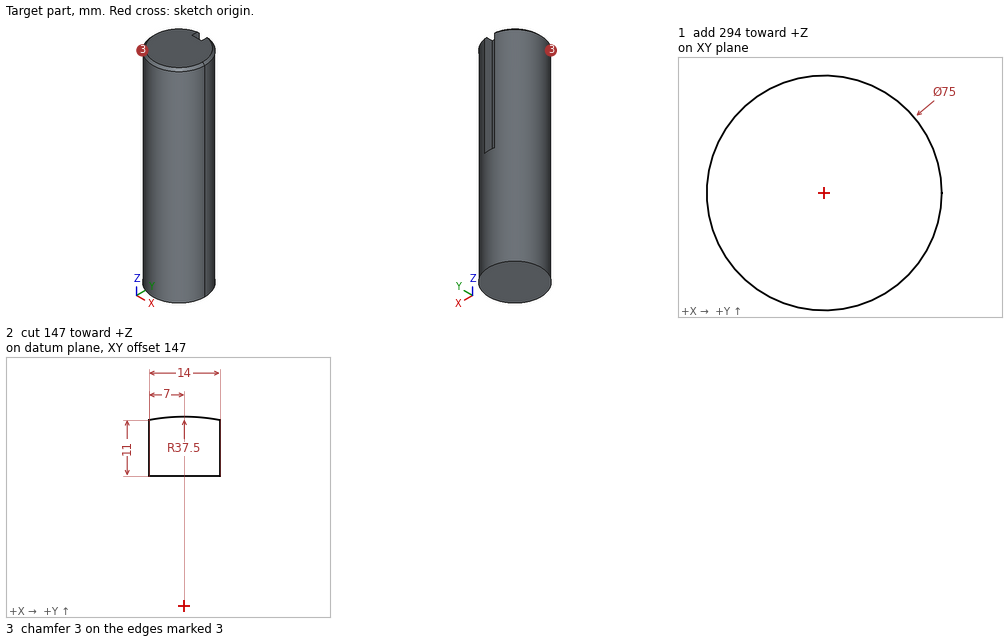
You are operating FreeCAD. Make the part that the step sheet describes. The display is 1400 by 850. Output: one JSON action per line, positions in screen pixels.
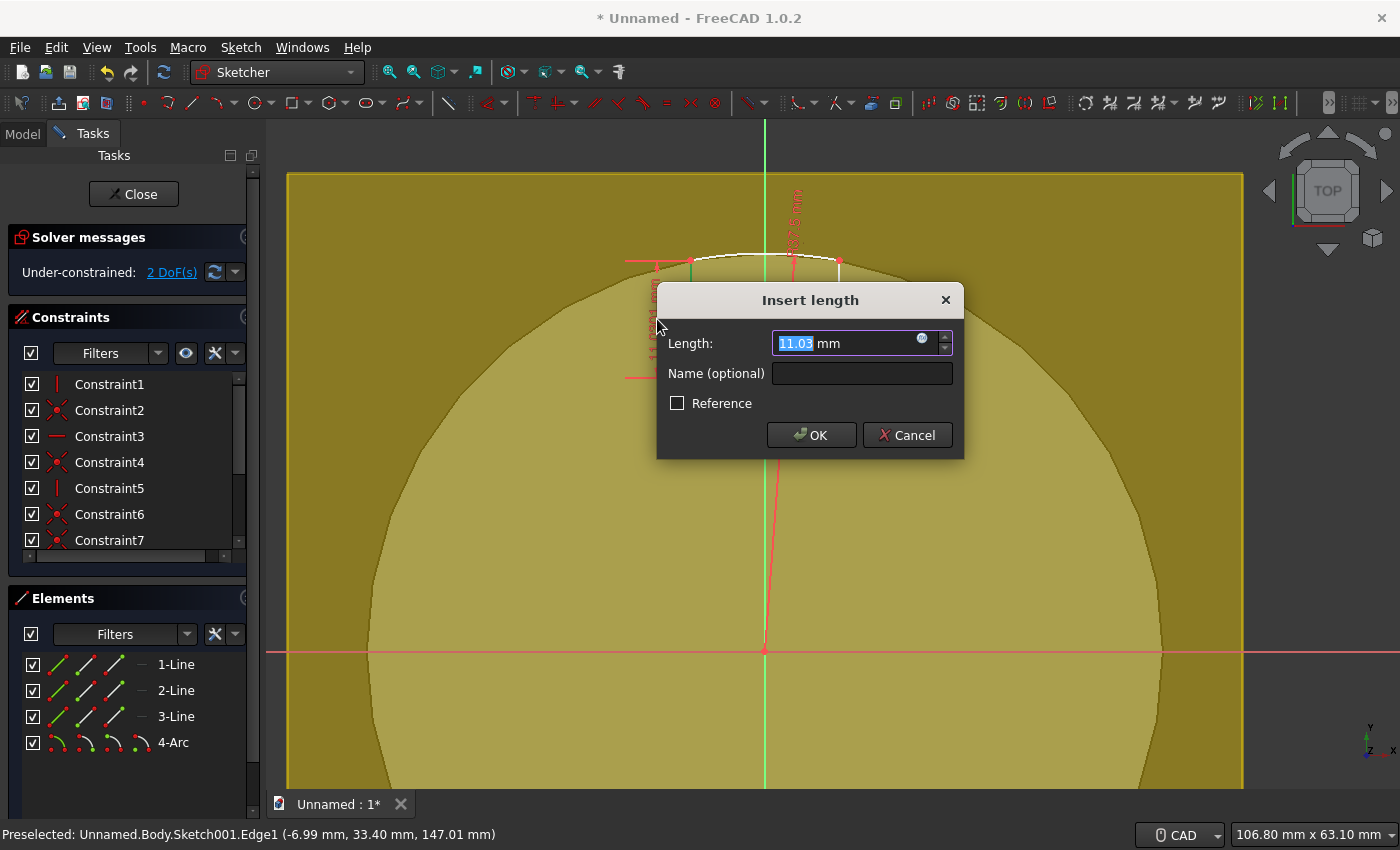
{"action": "type", "text": "11"}
{"action": "key", "text": "Return"}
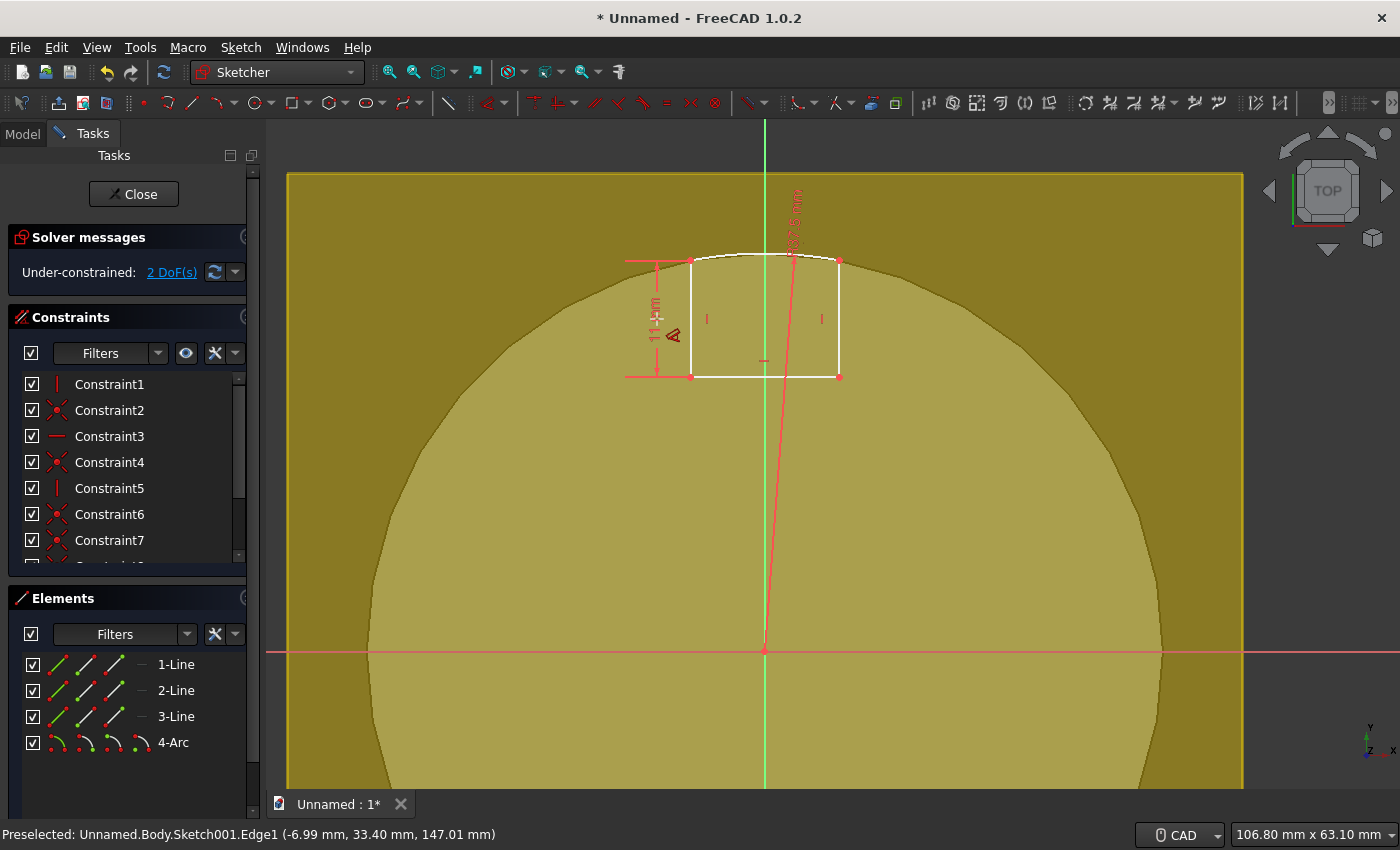
{"action": "left_click", "coordinate": [735, 377]}
{"action": "left_click", "coordinate": [731, 411]}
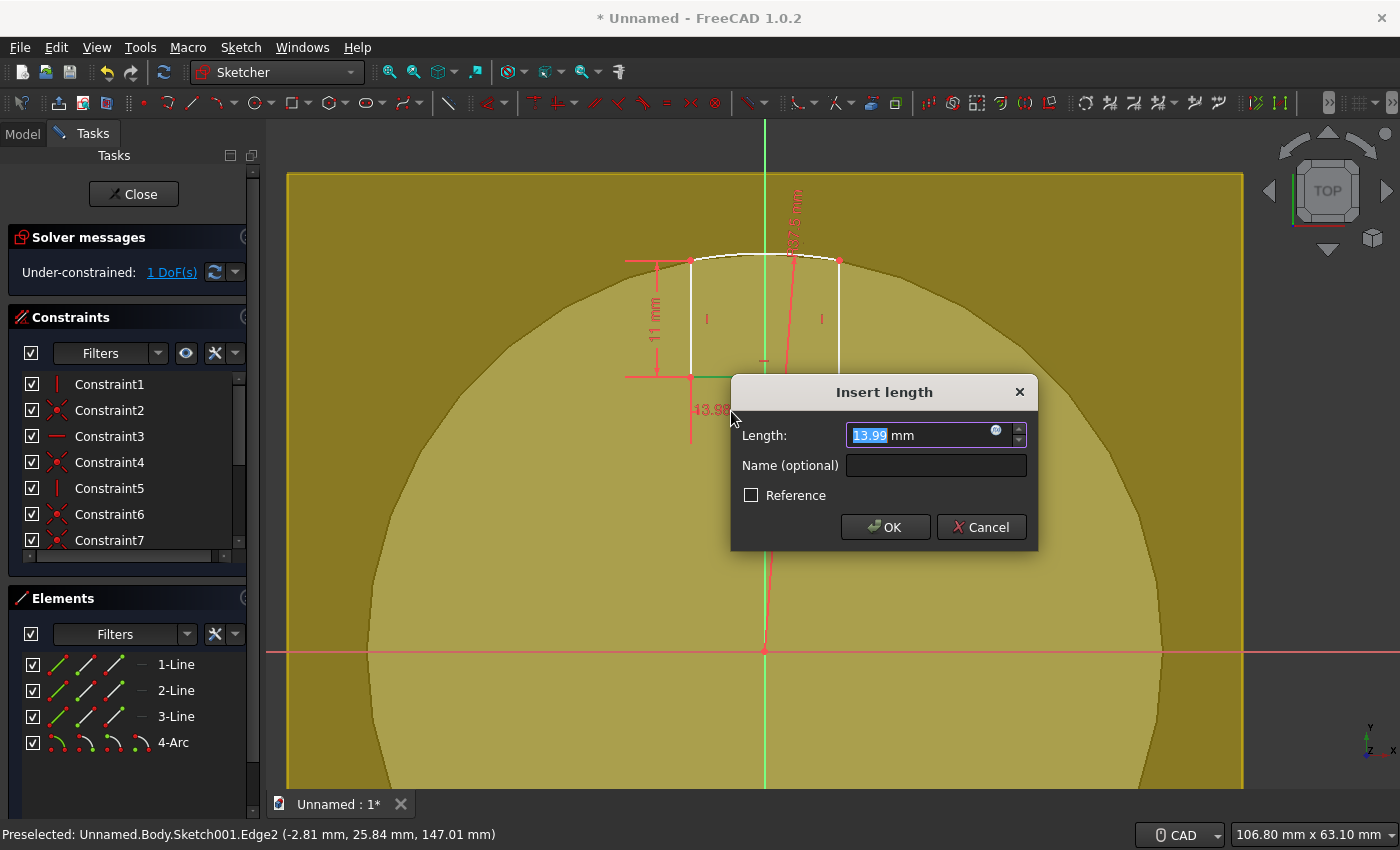
{"action": "type", "text": "14"}
{"action": "key", "text": "Return"}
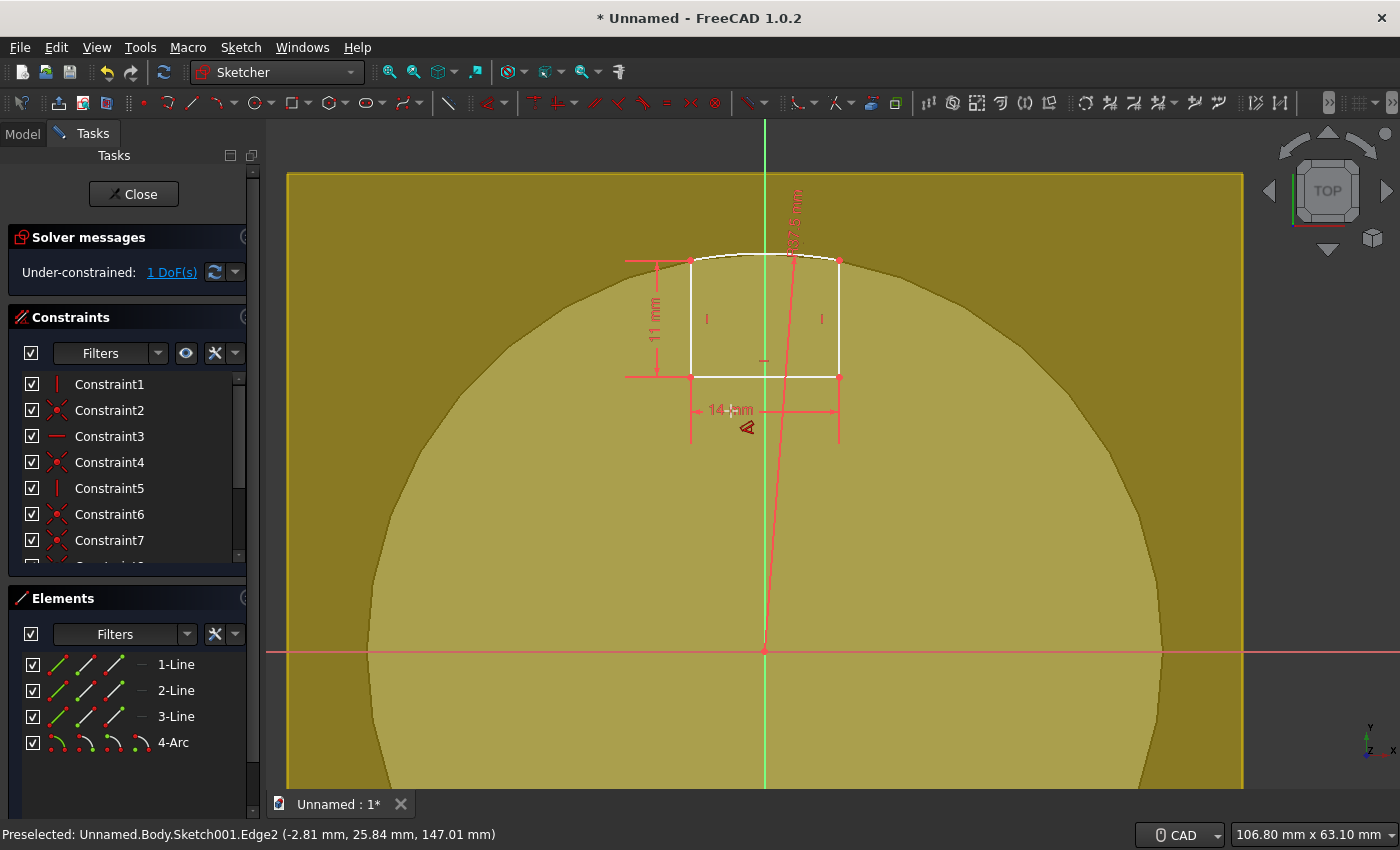
{"action": "left_click", "coordinate": [691, 260]}
{"action": "left_click", "coordinate": [728, 686]}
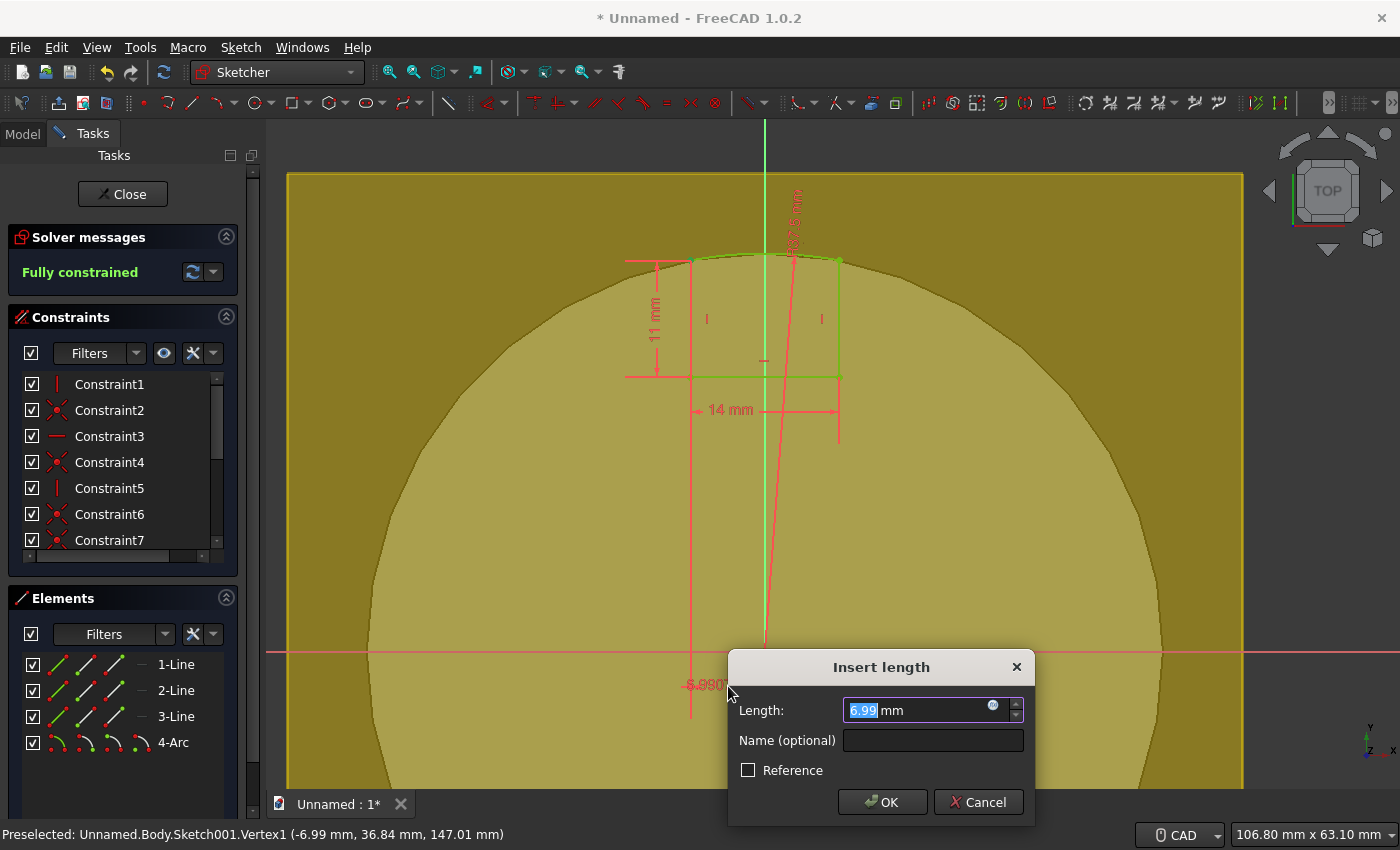
{"action": "type", "text": "7"}
{"action": "key", "text": "Return"}
{"action": "key", "text": "Escape"}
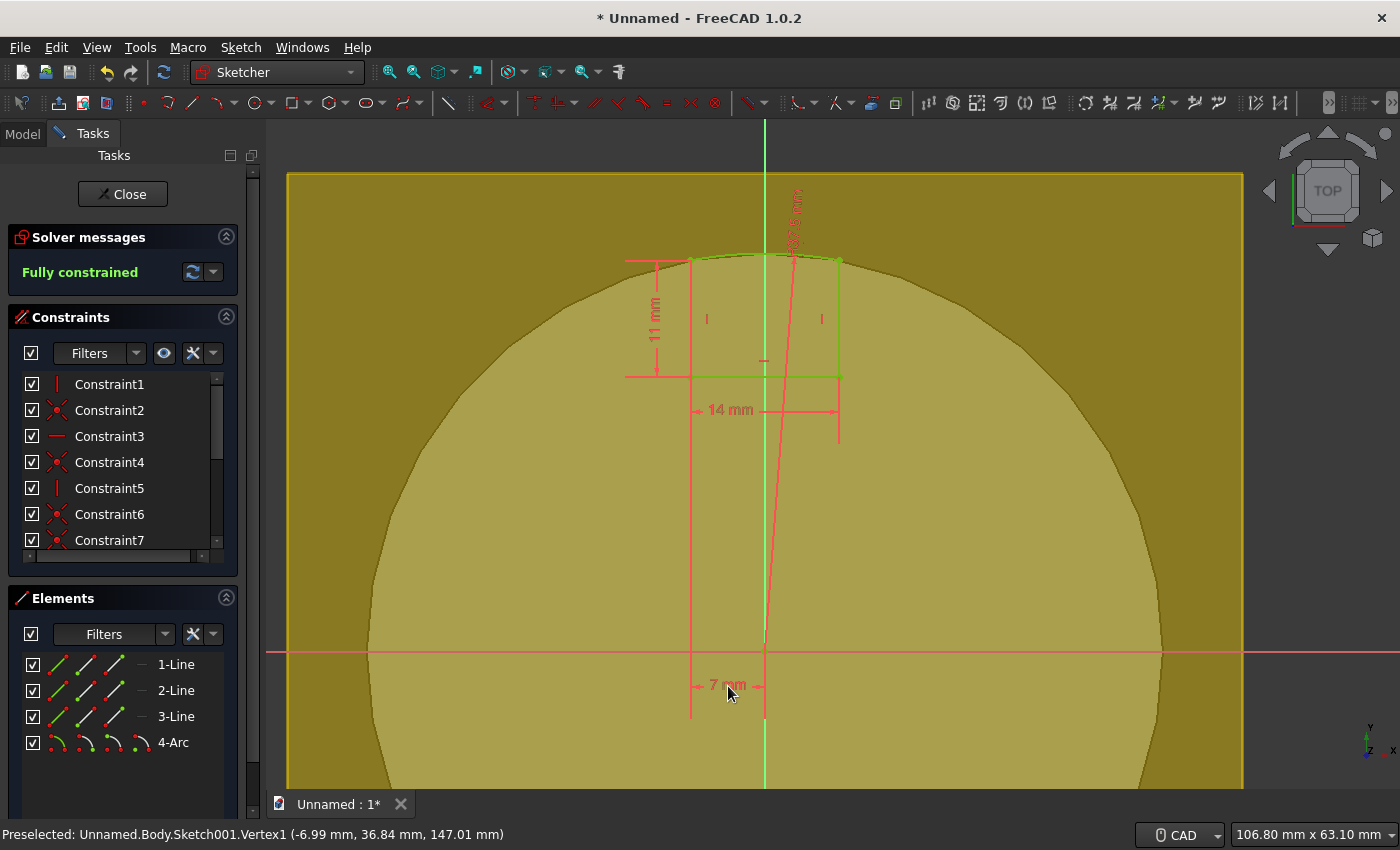
{"action": "left_click", "coordinate": [123, 194]}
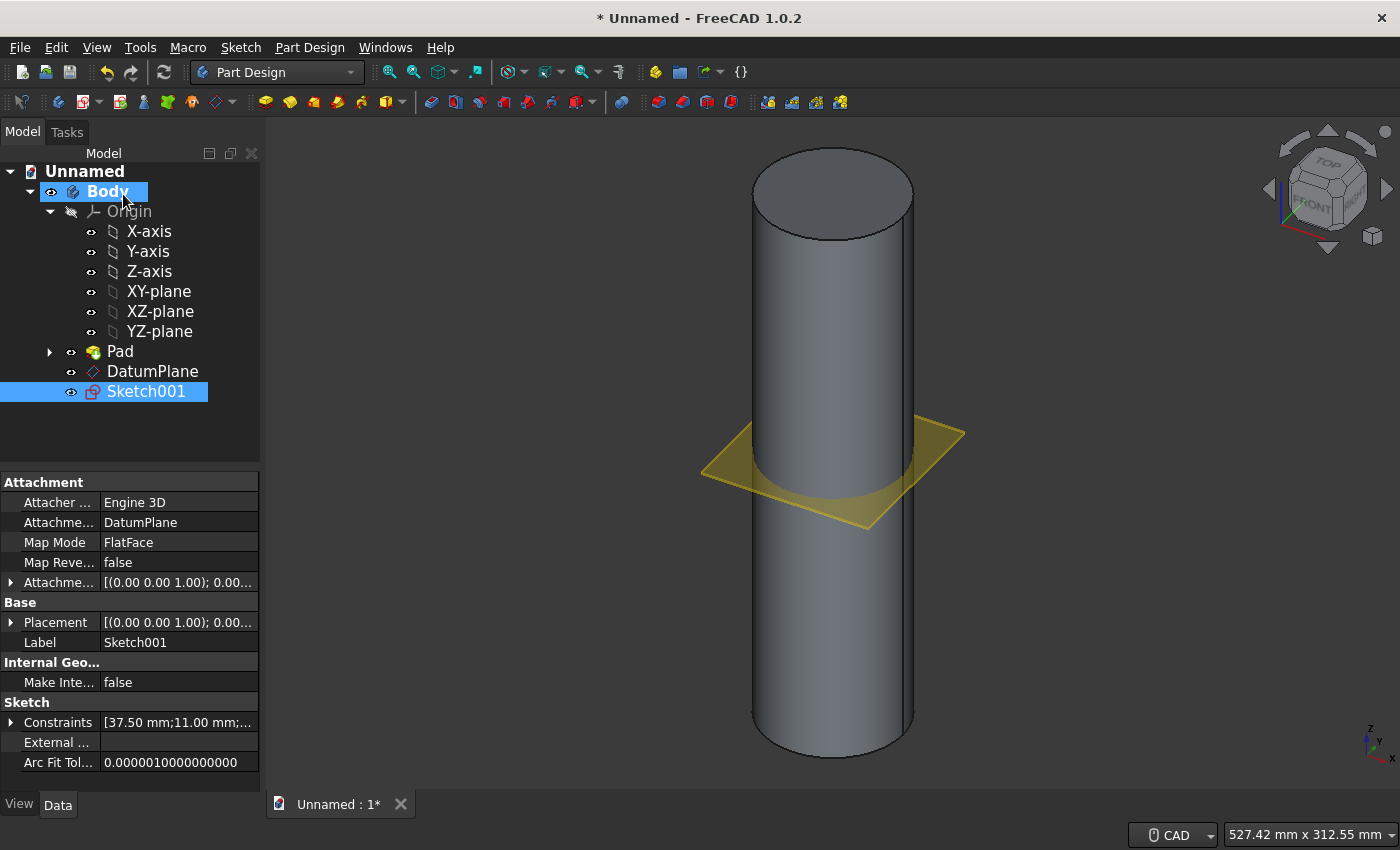
{"action": "left_click", "coordinate": [432, 102]}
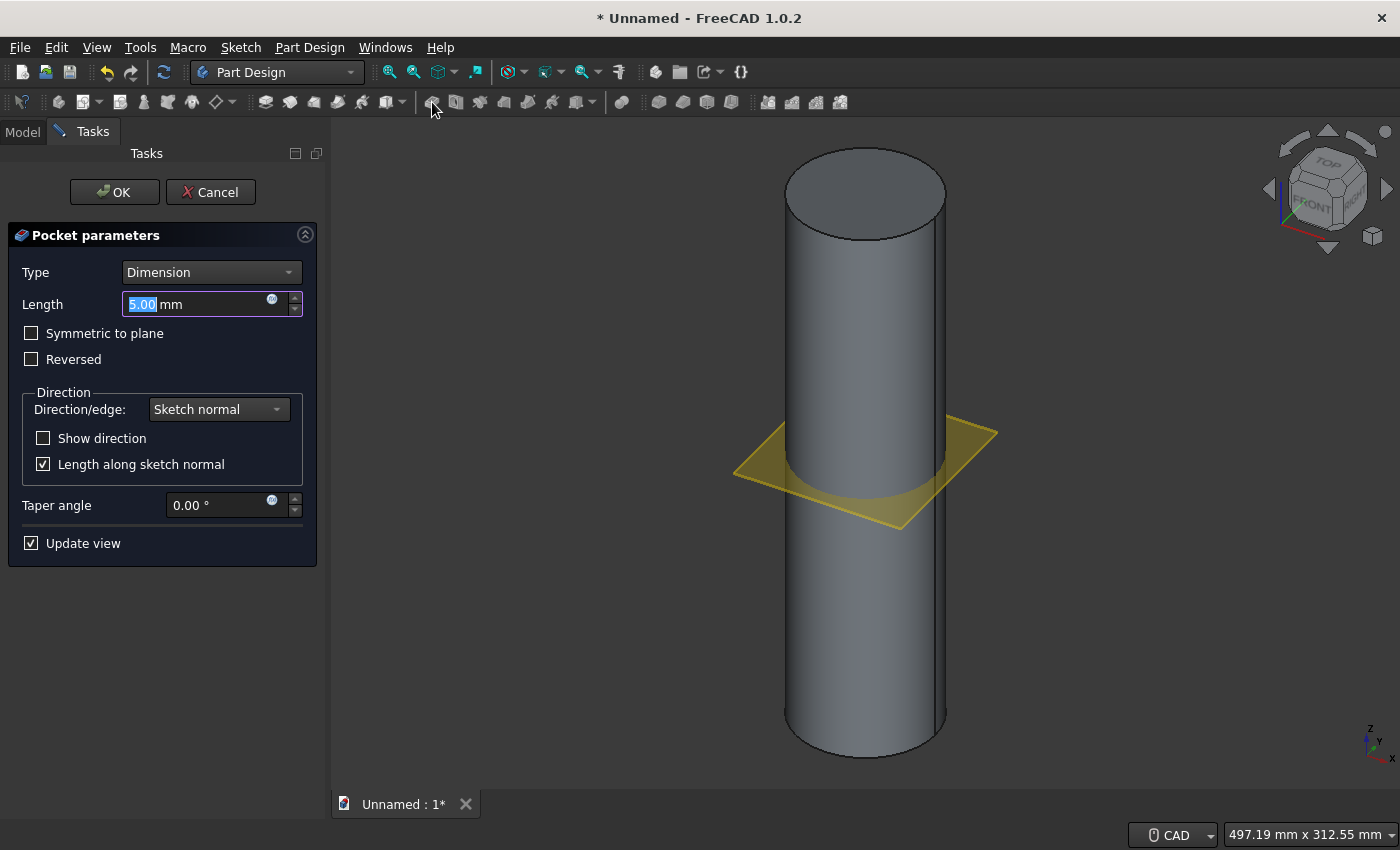
{"action": "type", "text": "147"}
{"action": "key", "text": "Tab"}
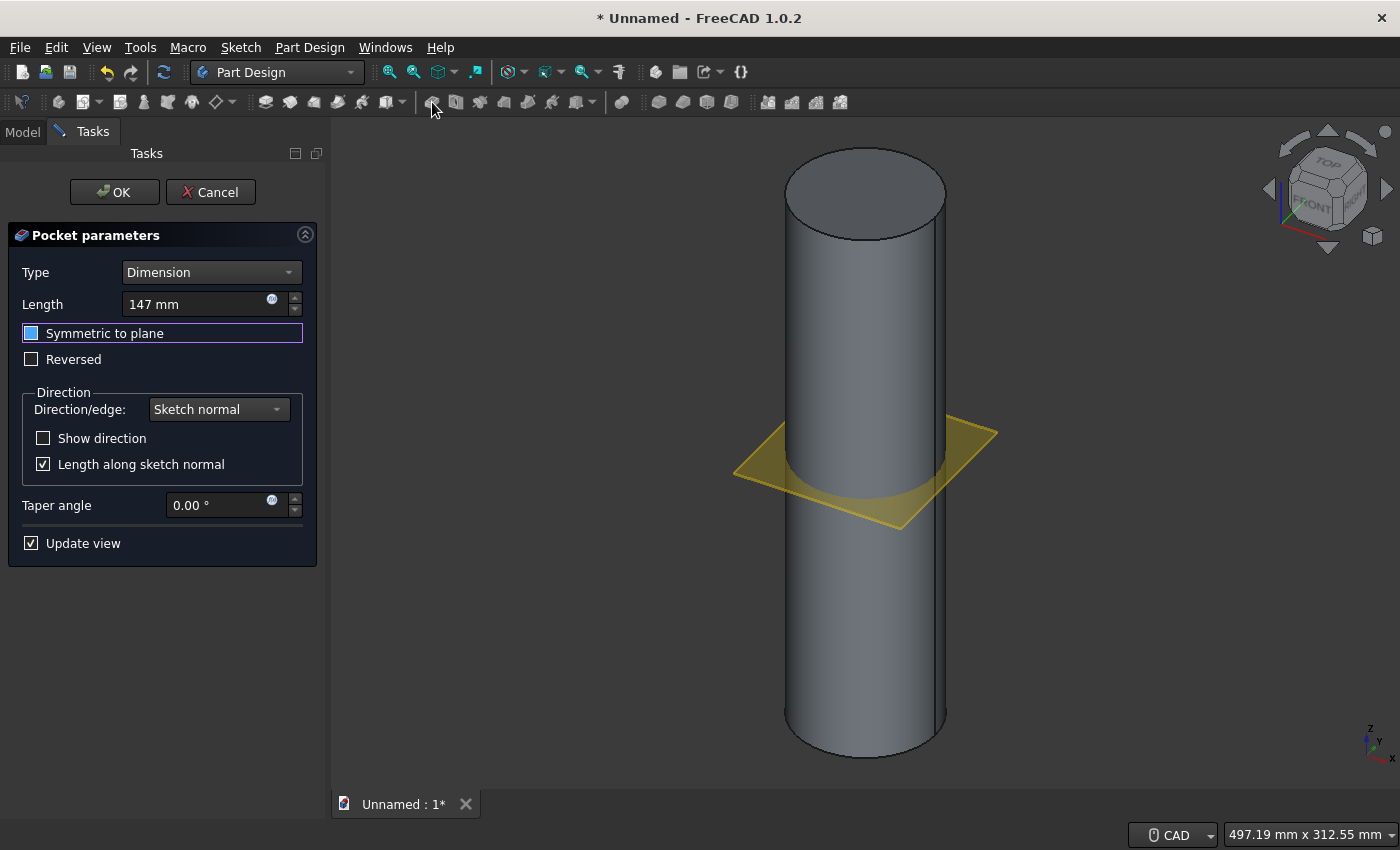
{"action": "left_click", "coordinate": [30, 359]}